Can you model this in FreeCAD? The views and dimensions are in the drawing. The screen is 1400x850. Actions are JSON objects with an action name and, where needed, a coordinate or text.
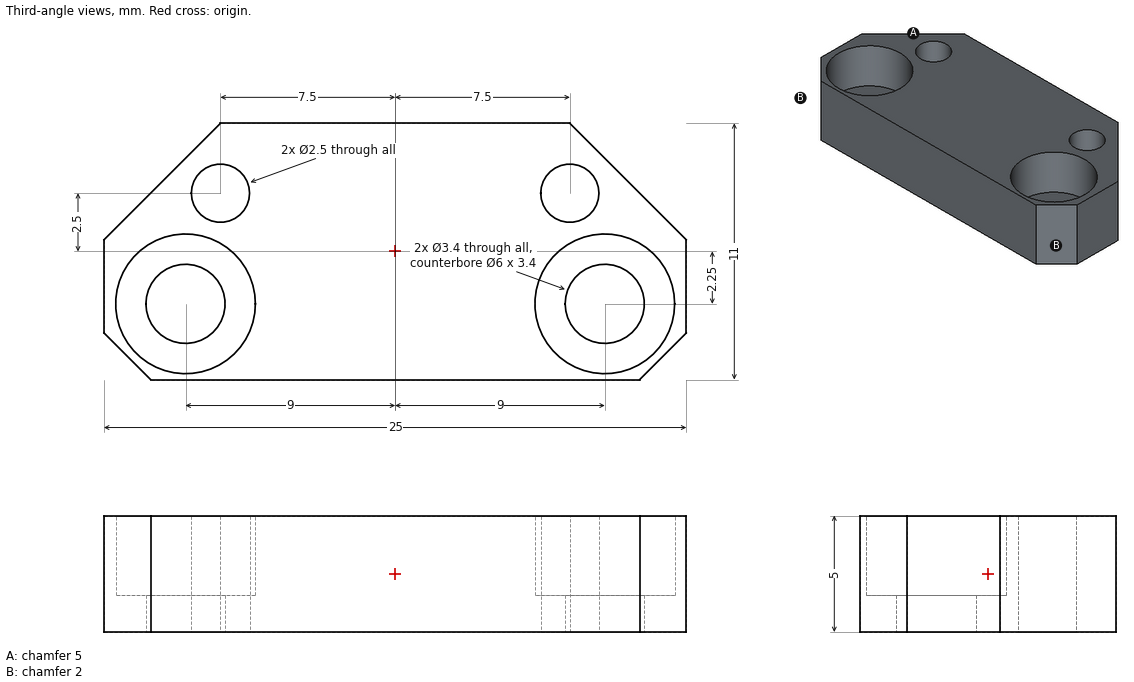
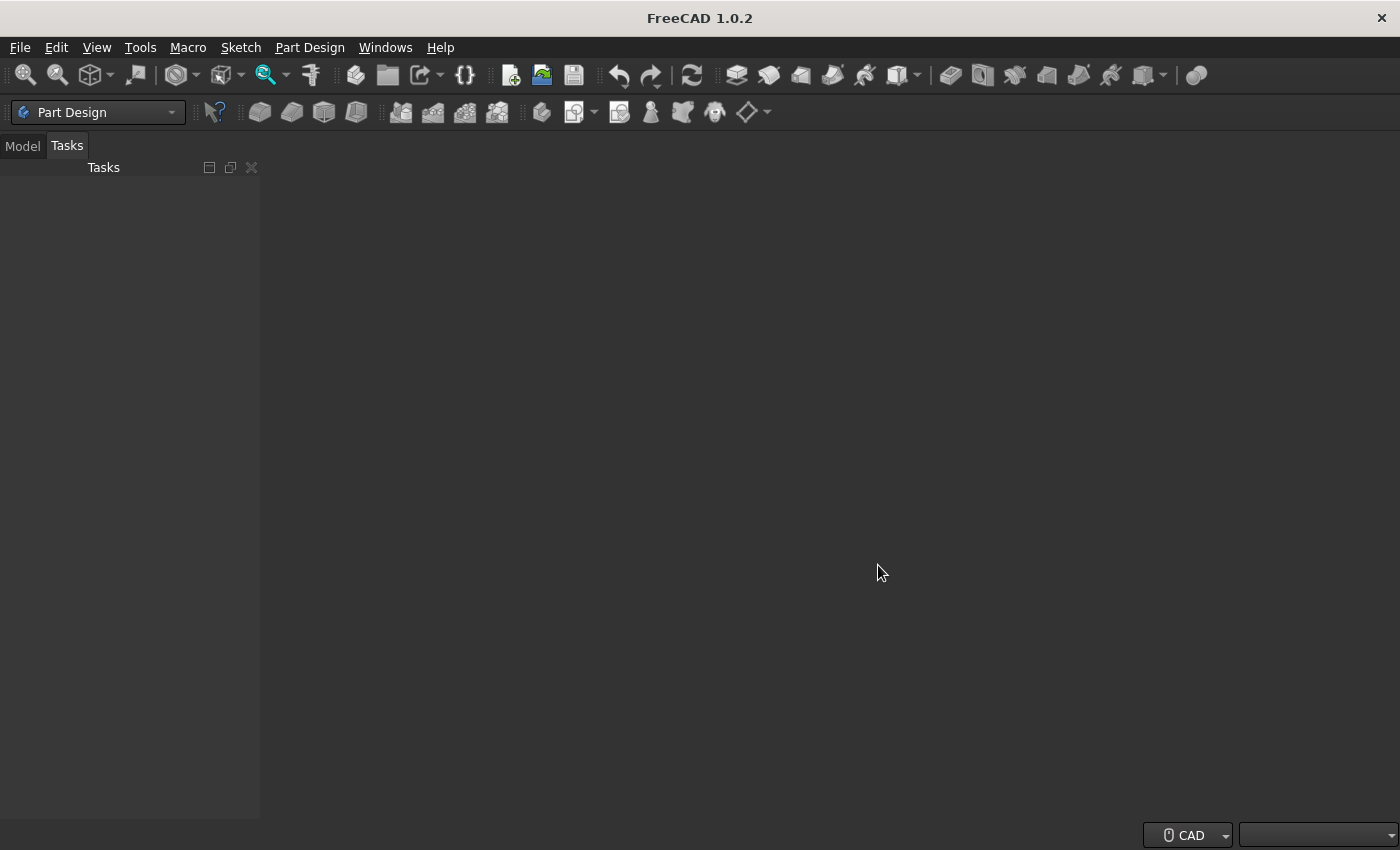
{"action": "key", "text": "ctrl+n"}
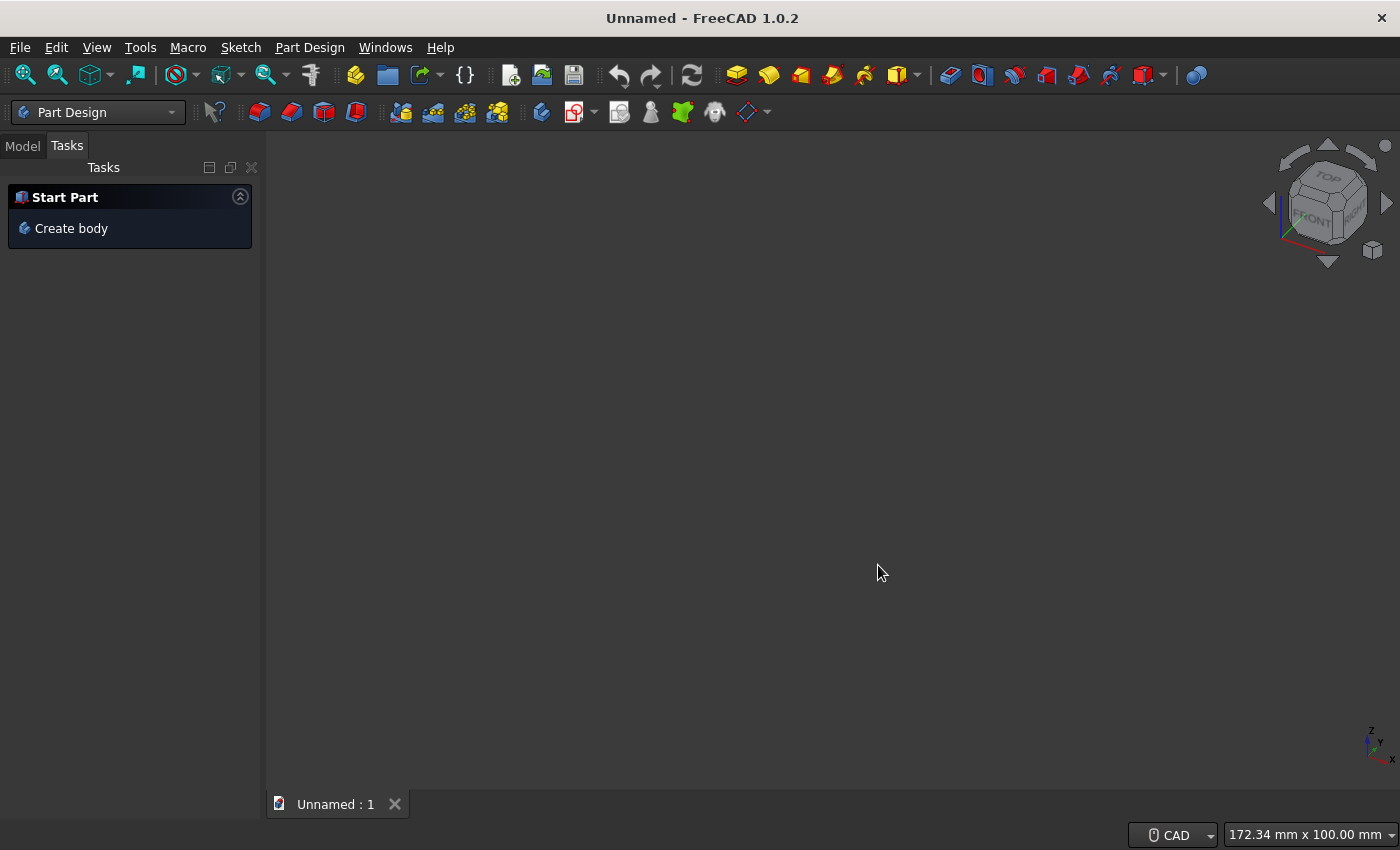
{"action": "left_click", "coordinate": [574, 112]}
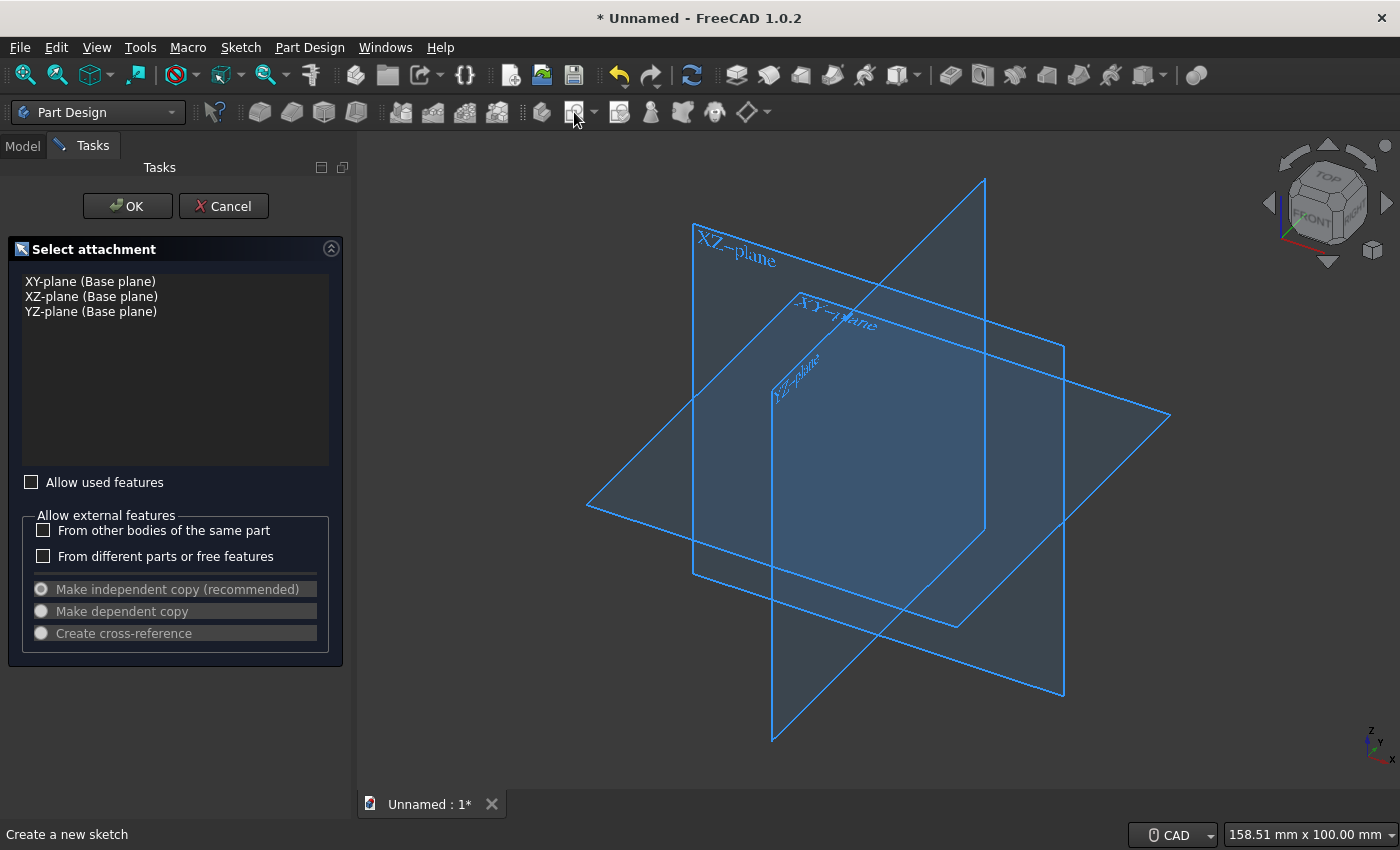
{"action": "left_click", "coordinate": [82, 282]}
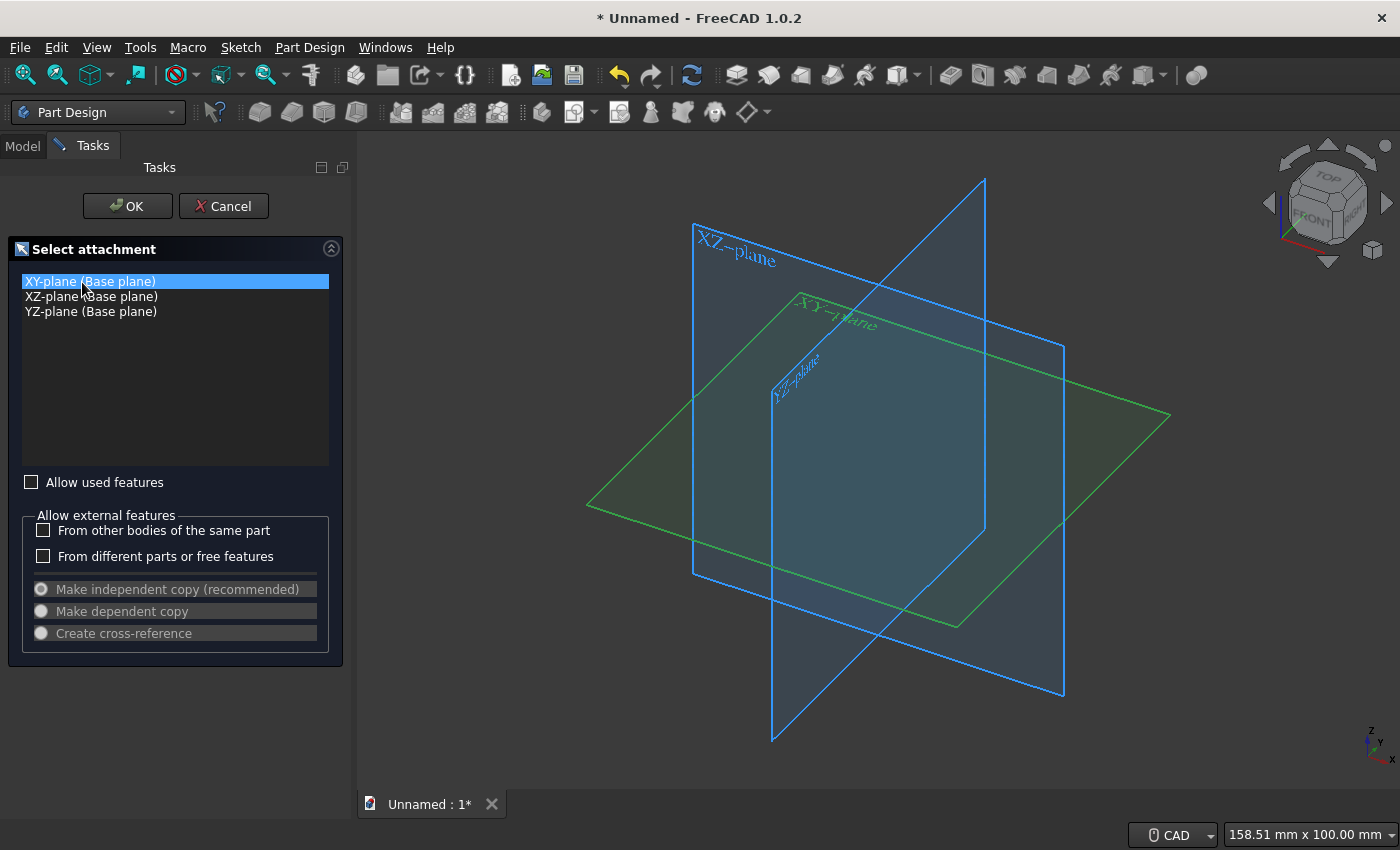
{"action": "left_click", "coordinate": [128, 206]}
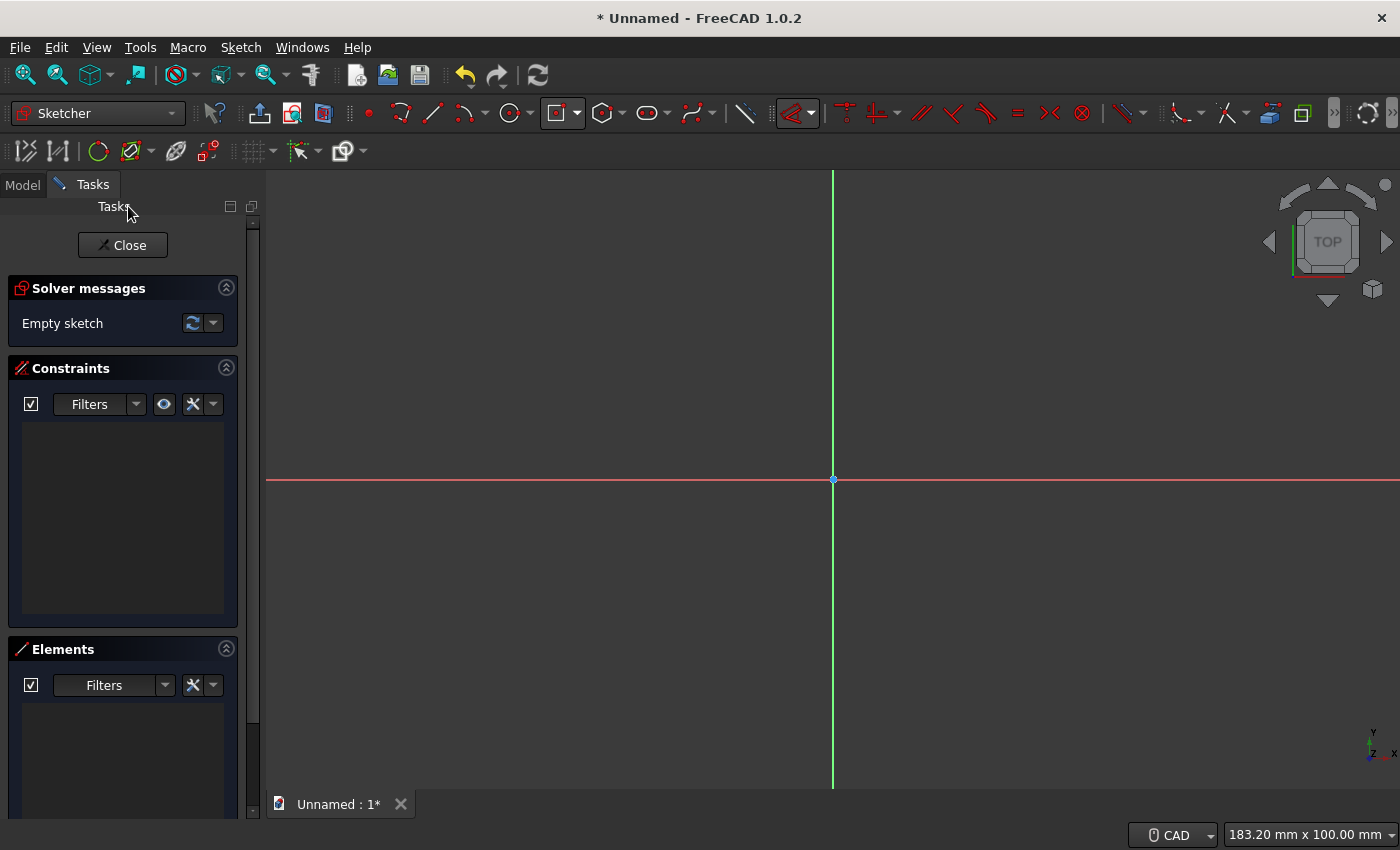
{"action": "scroll", "coordinate": [855, 480], "scroll_direction": "up", "scroll_amount": 7}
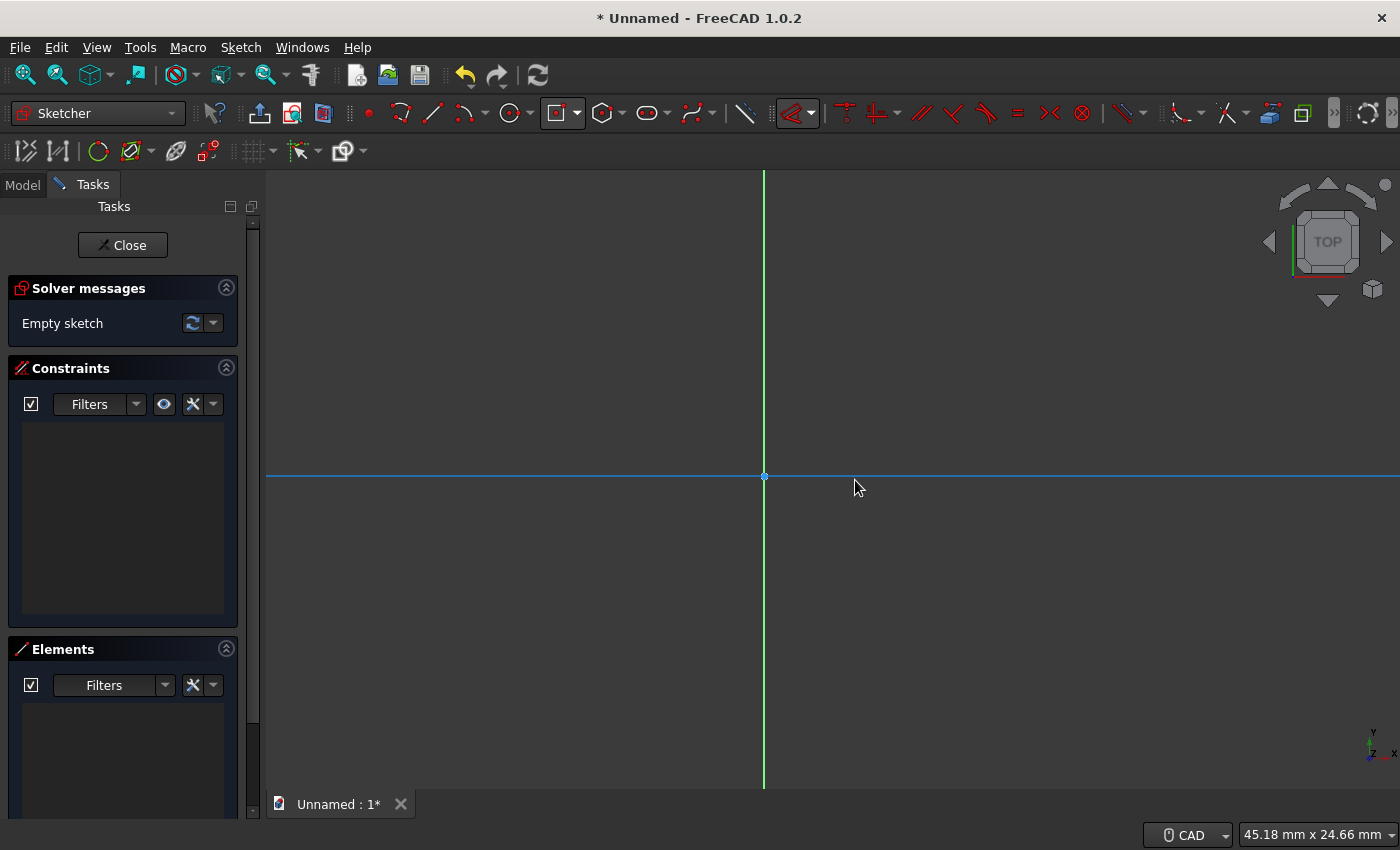
{"action": "left_click", "coordinate": [556, 114]}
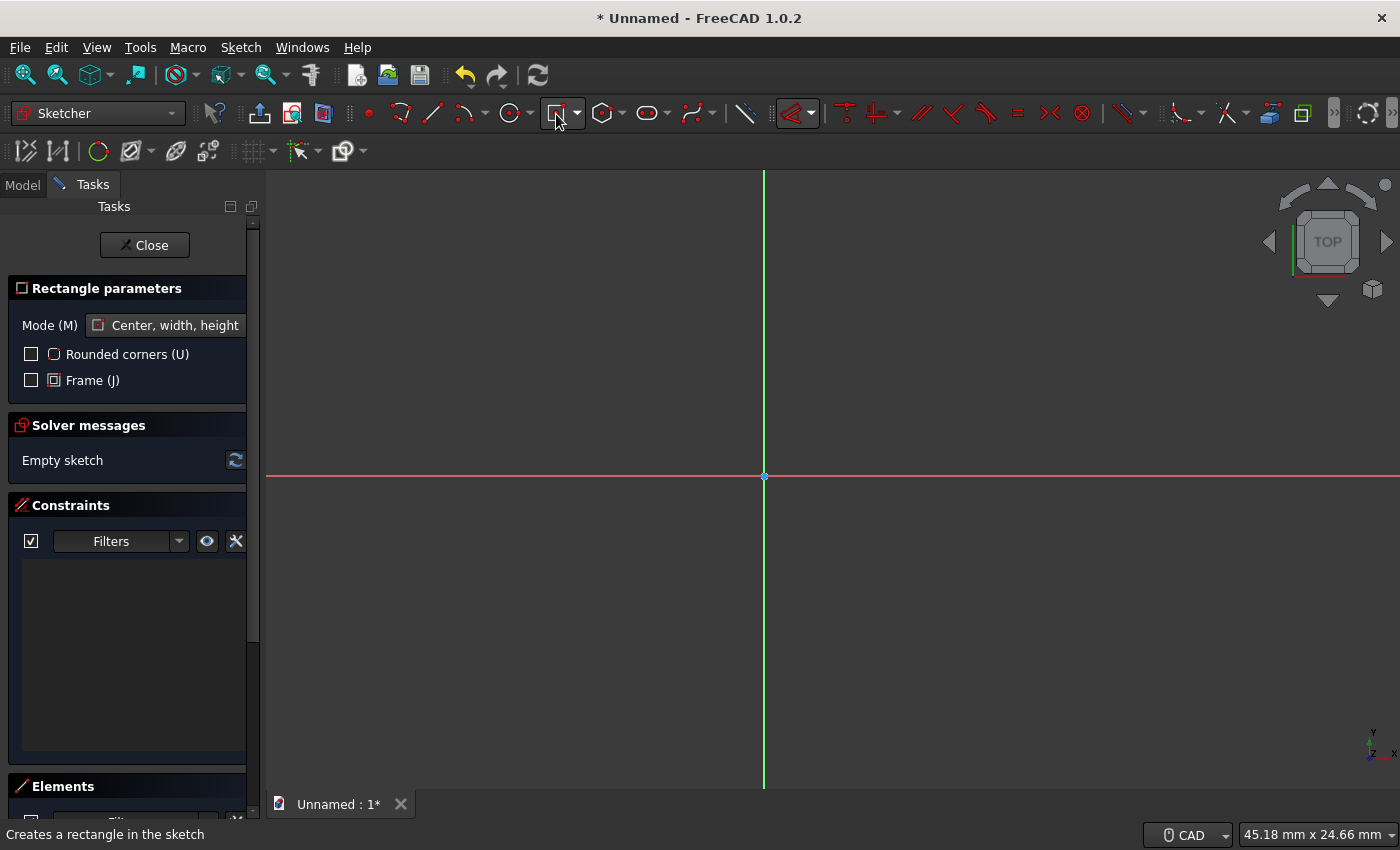
{"action": "left_click", "coordinate": [764, 476]}
{"action": "left_click", "coordinate": [1078, 338]}
{"action": "key", "text": "Escape"}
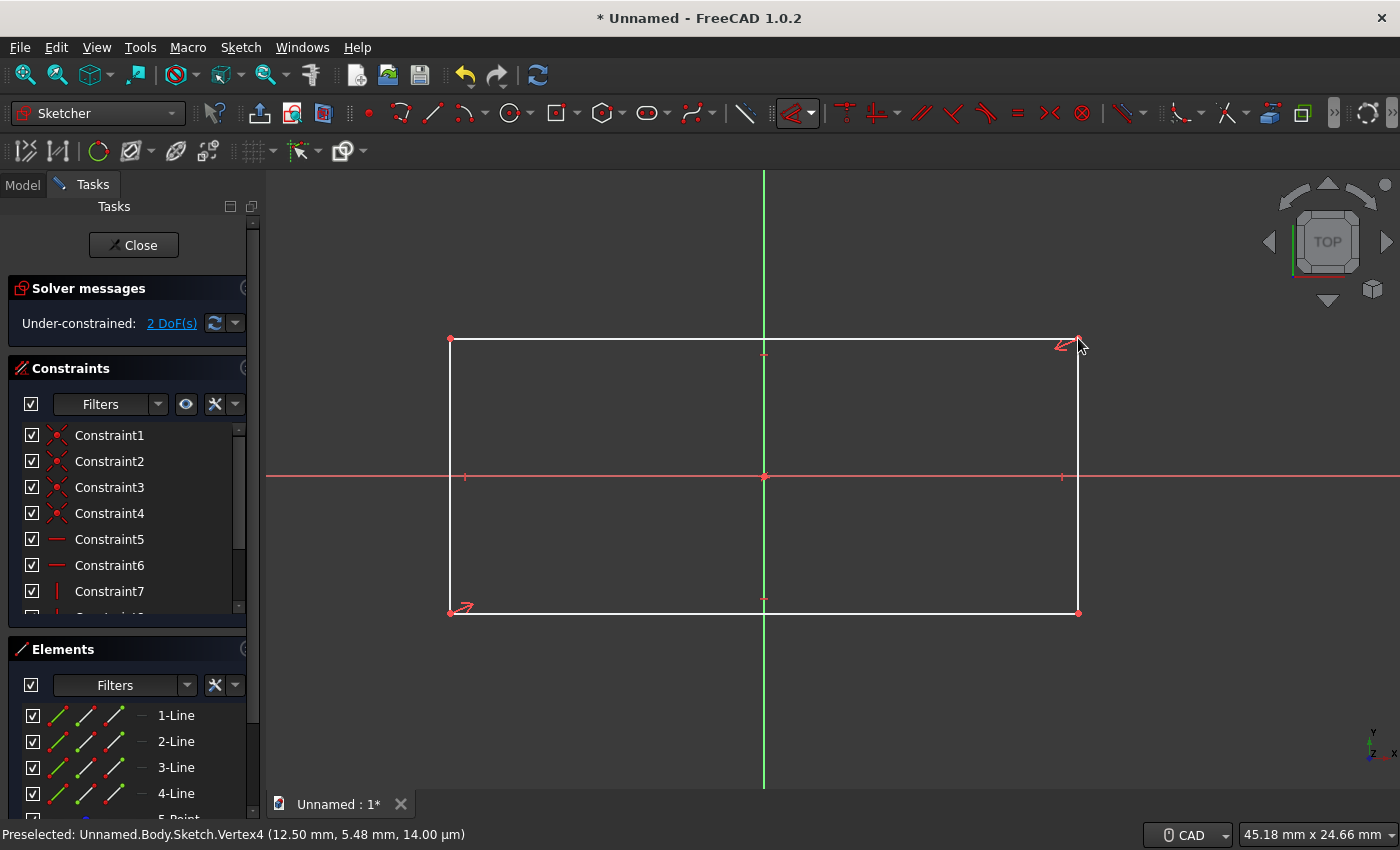
{"action": "left_click", "coordinate": [792, 114]}